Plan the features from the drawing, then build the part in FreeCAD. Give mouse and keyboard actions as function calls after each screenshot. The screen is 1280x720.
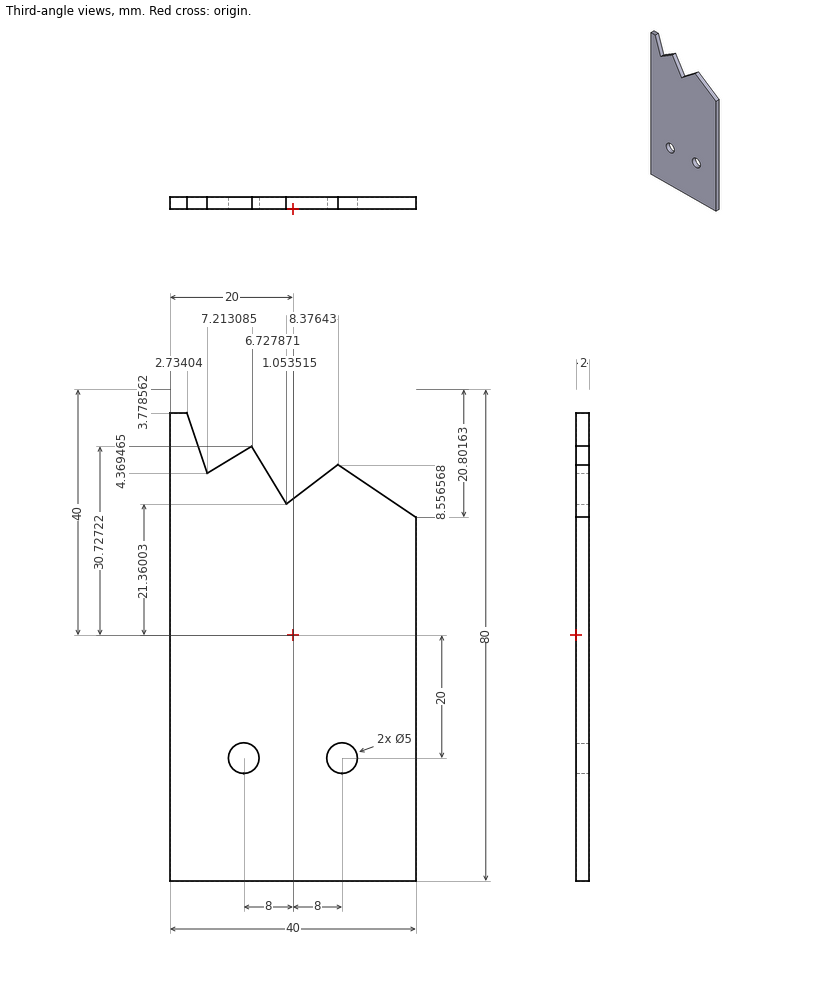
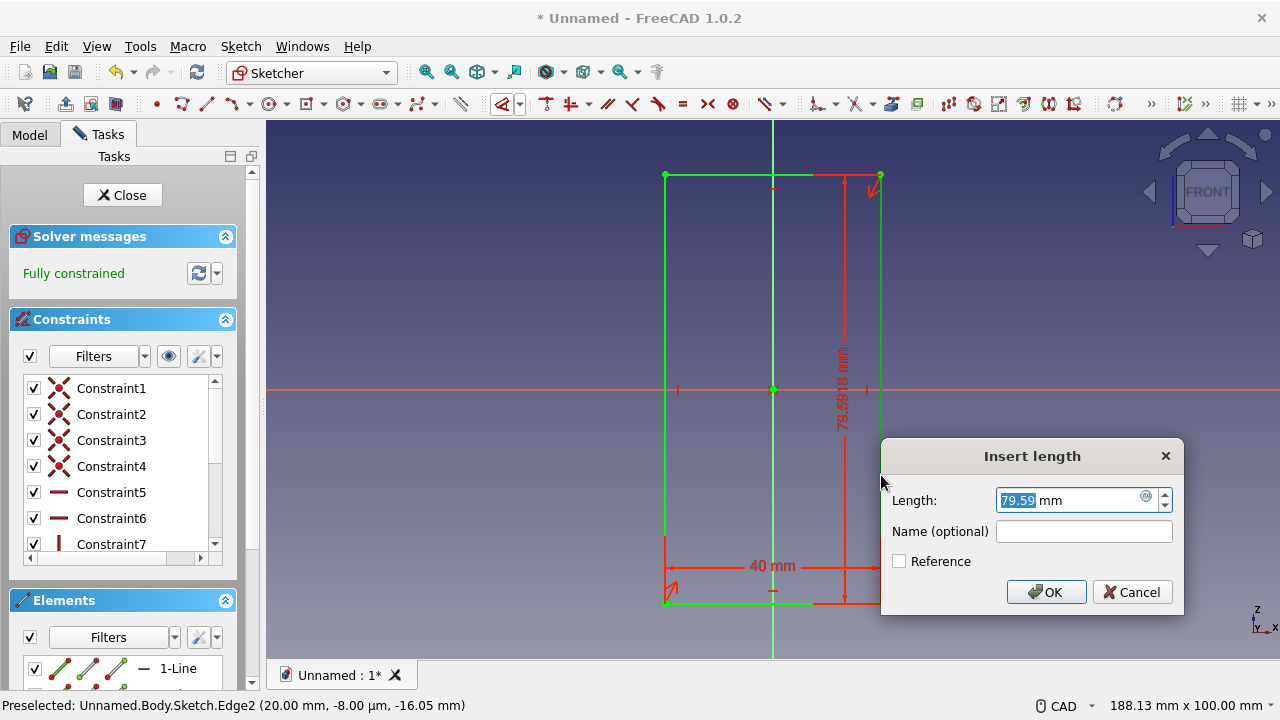
text(80)
key(Return)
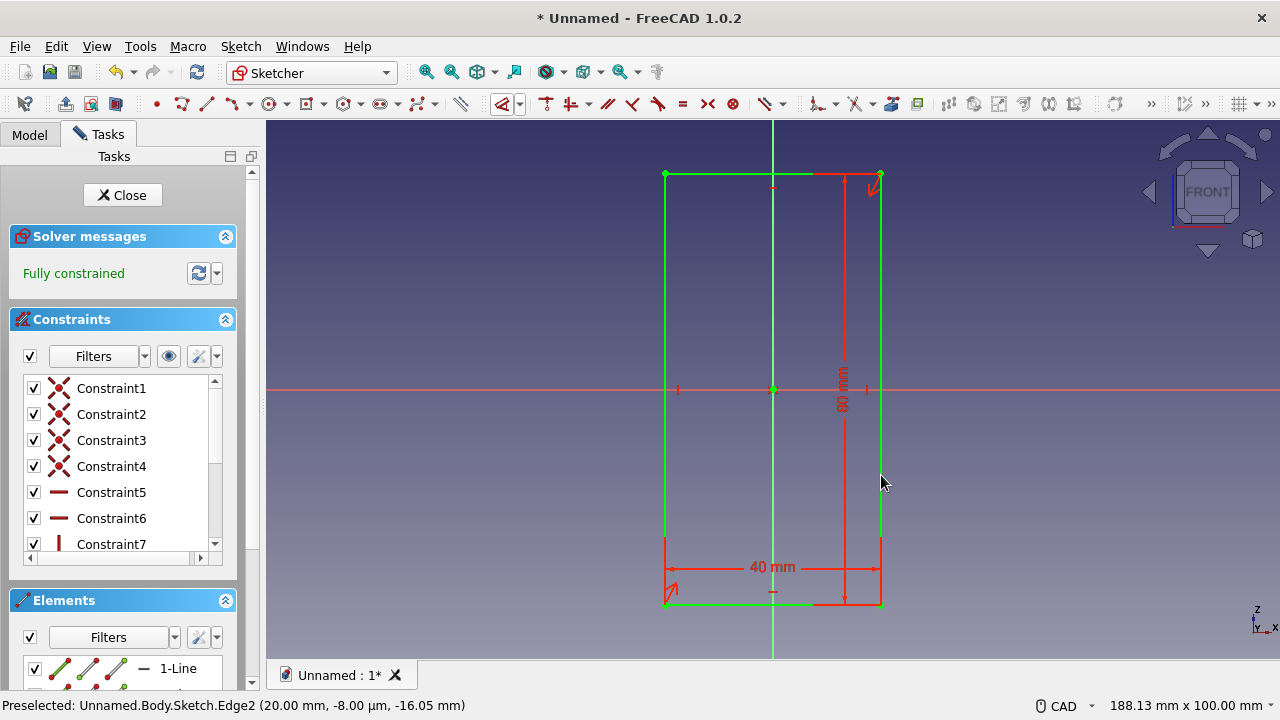
click(123, 195)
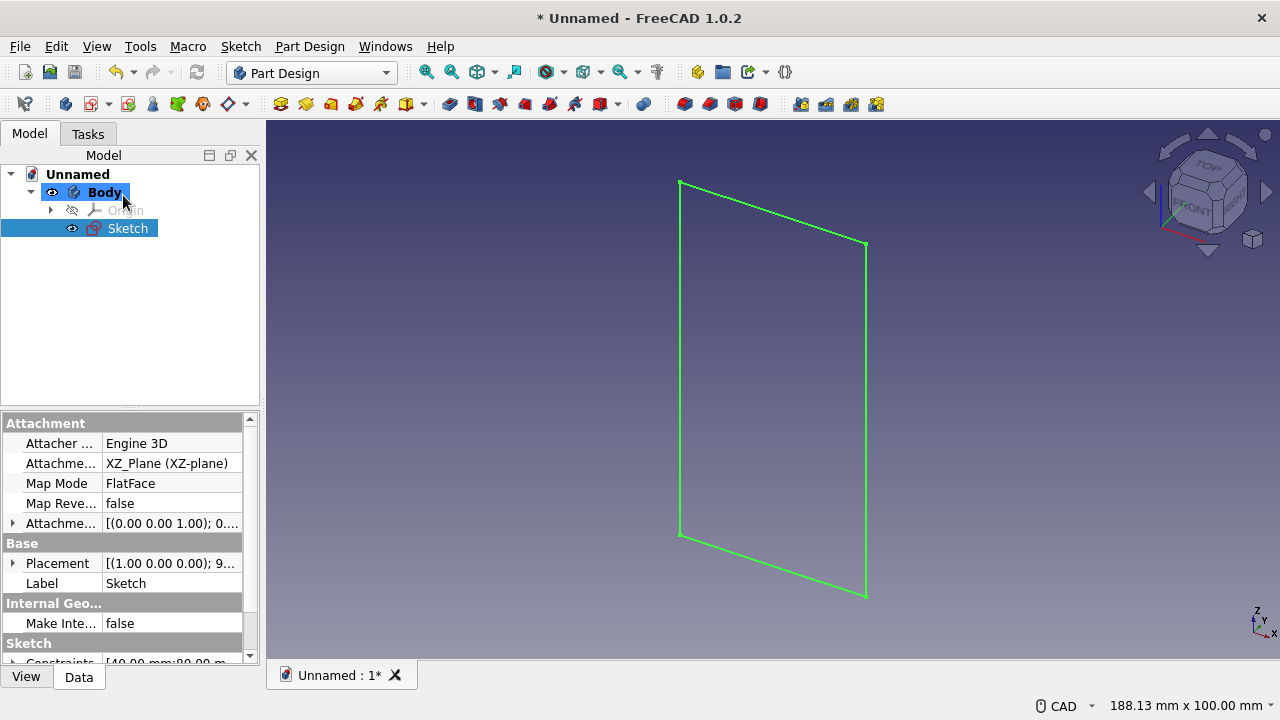
click(281, 104)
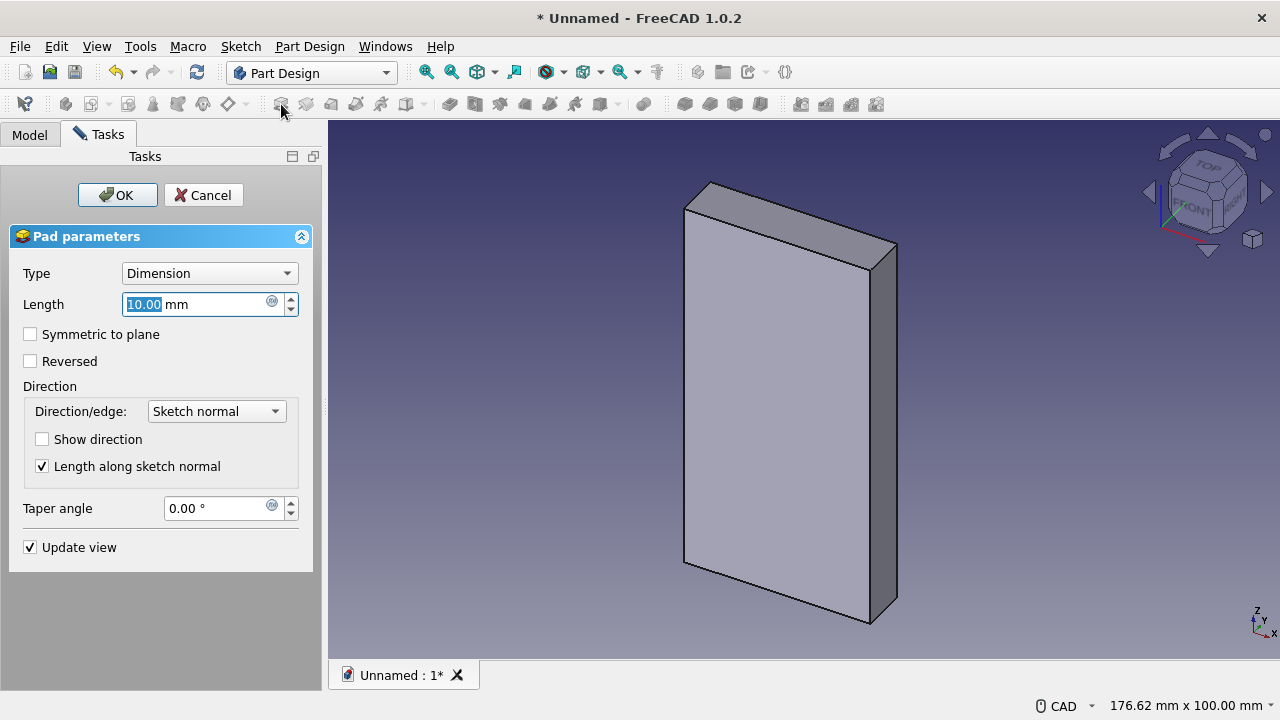
text(2)
key(Tab)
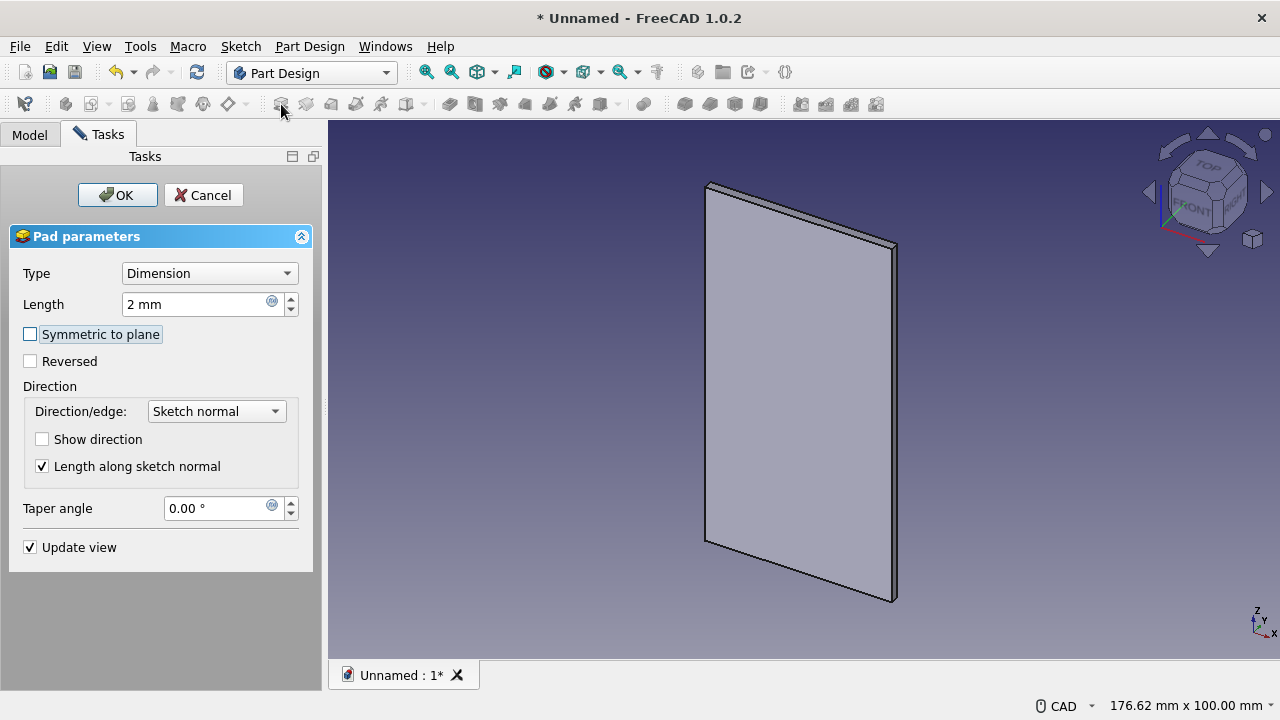
click(31, 361)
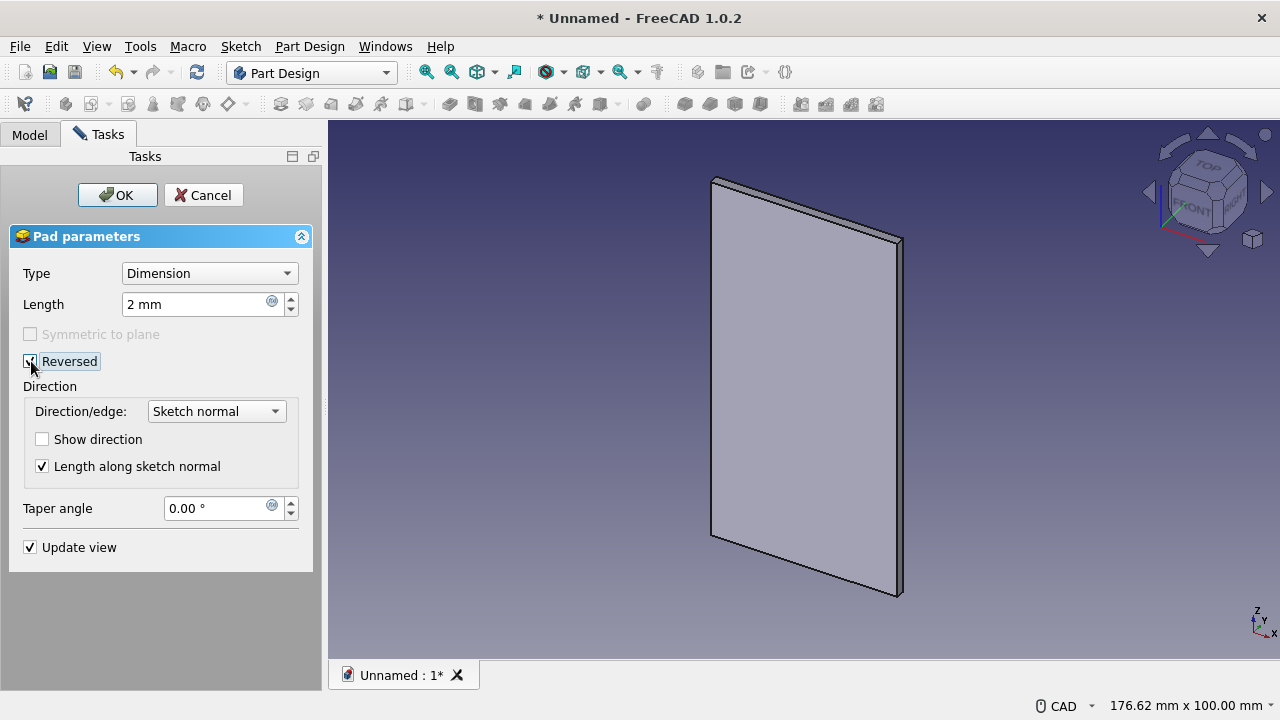
click(118, 195)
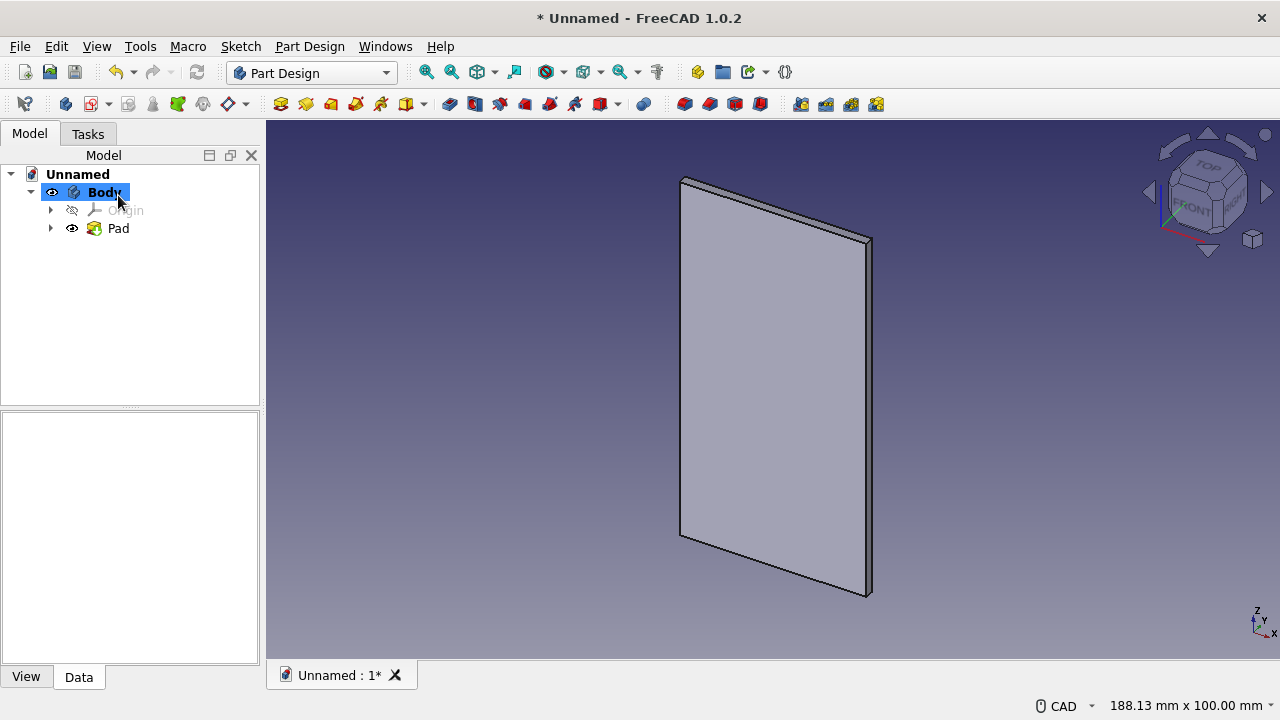
click(90, 104)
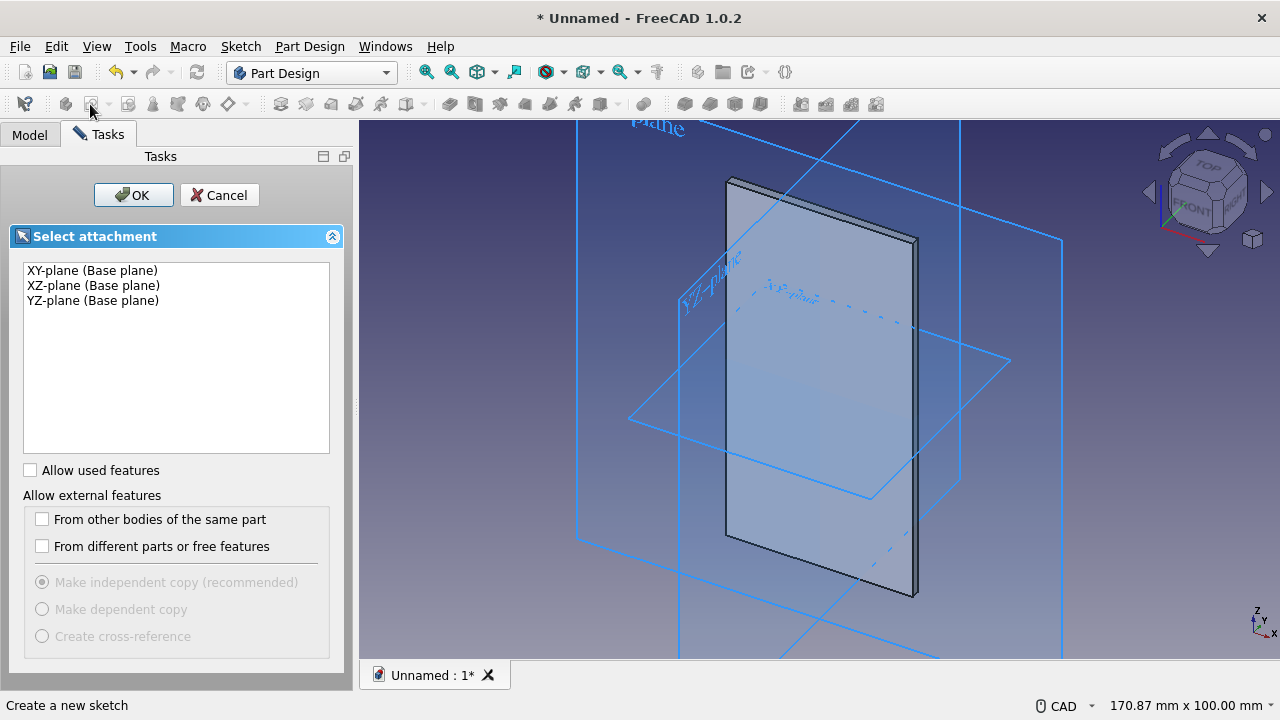
click(84, 286)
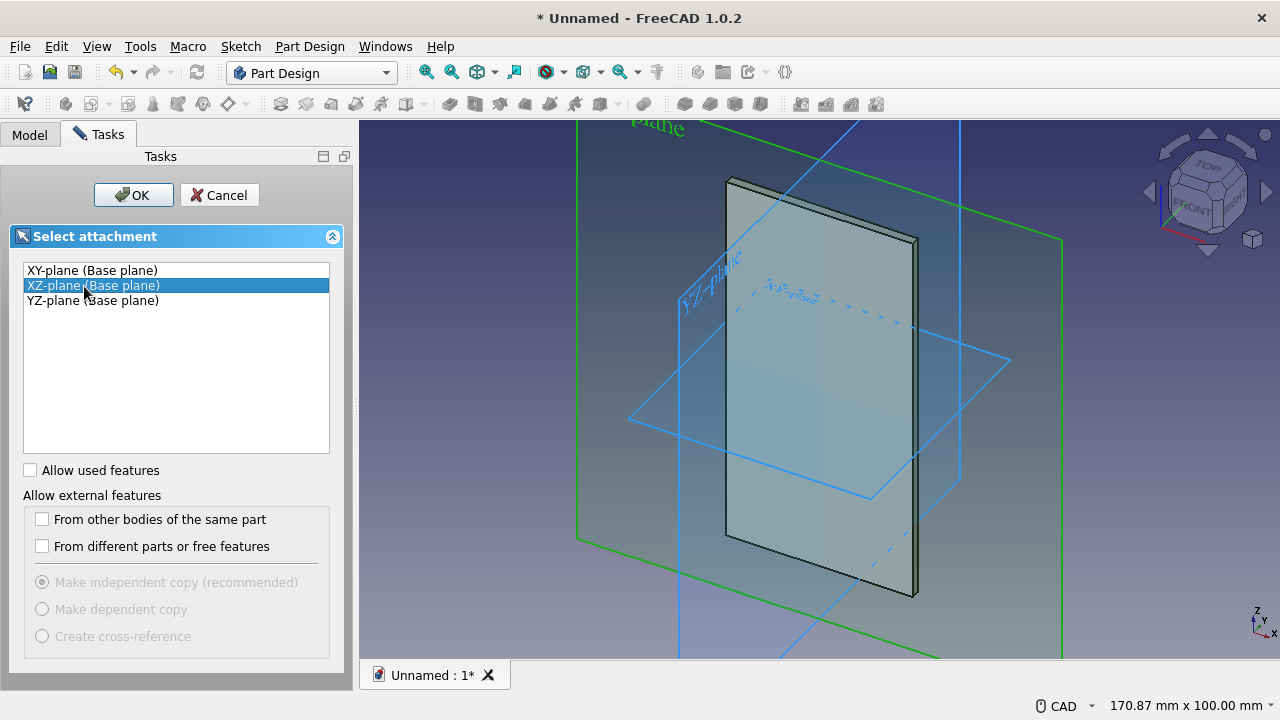
click(134, 195)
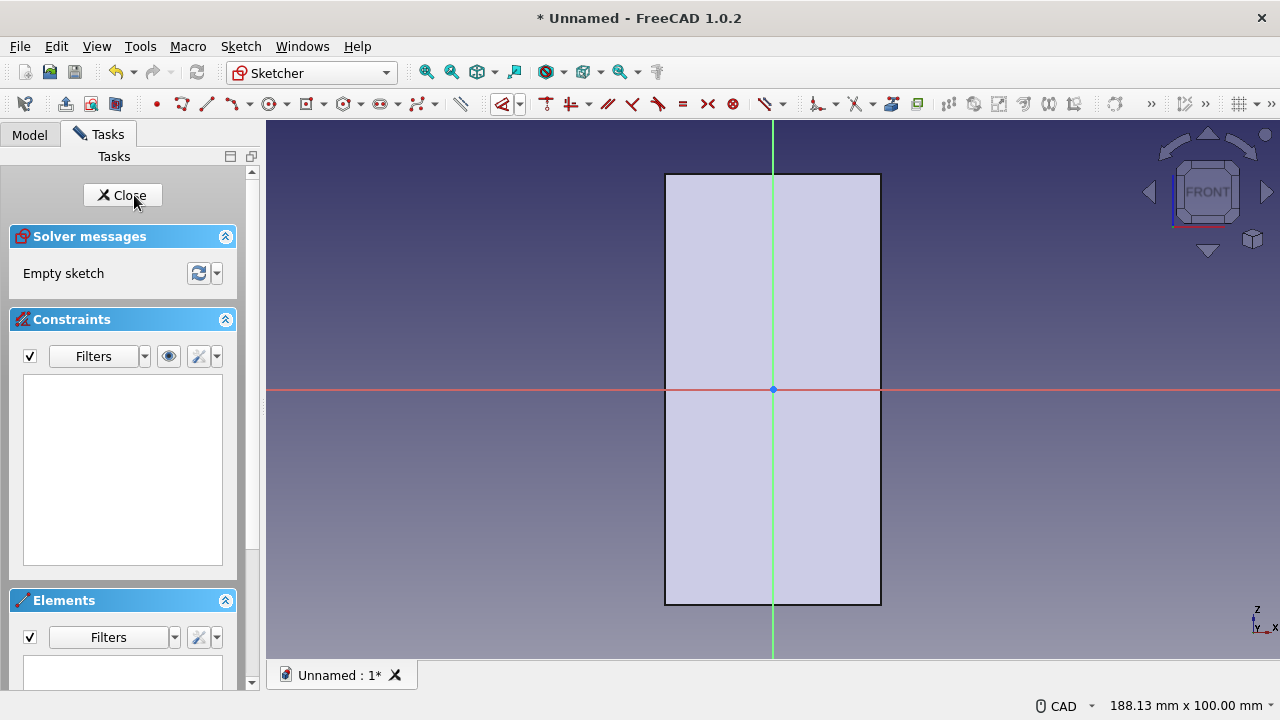
scroll(813, 485, up, 5)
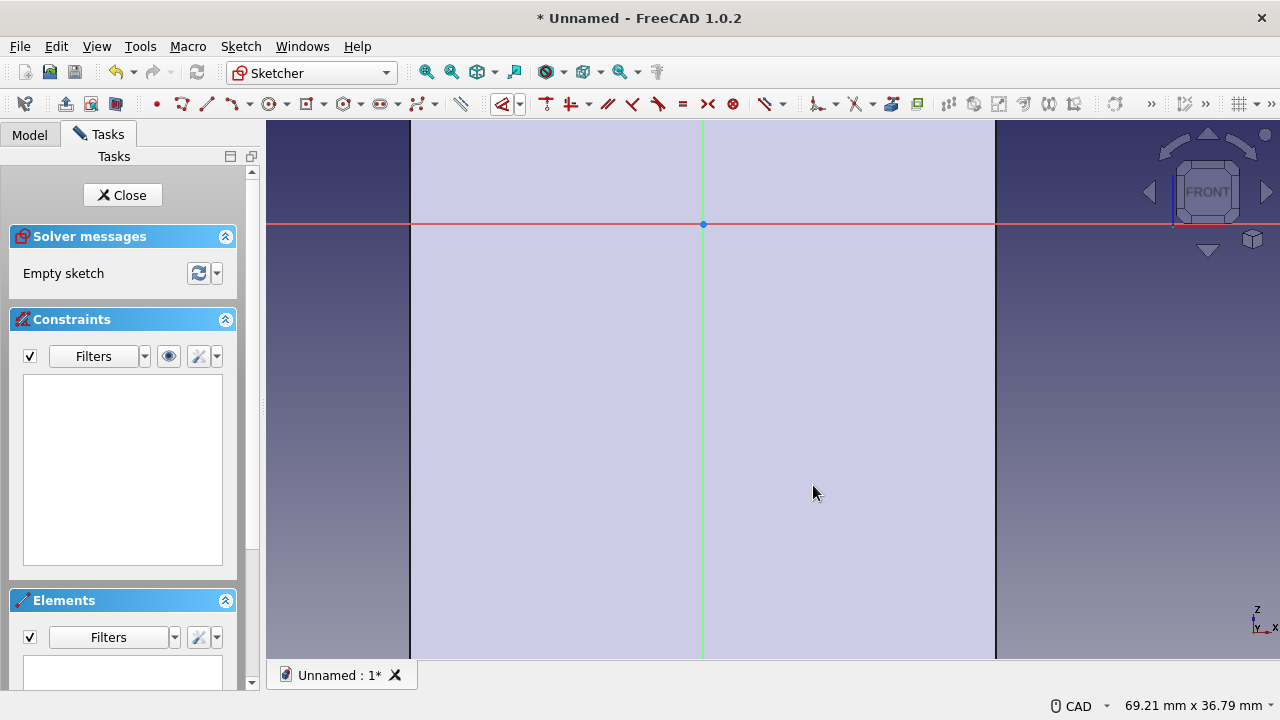
key(g)
key(c)